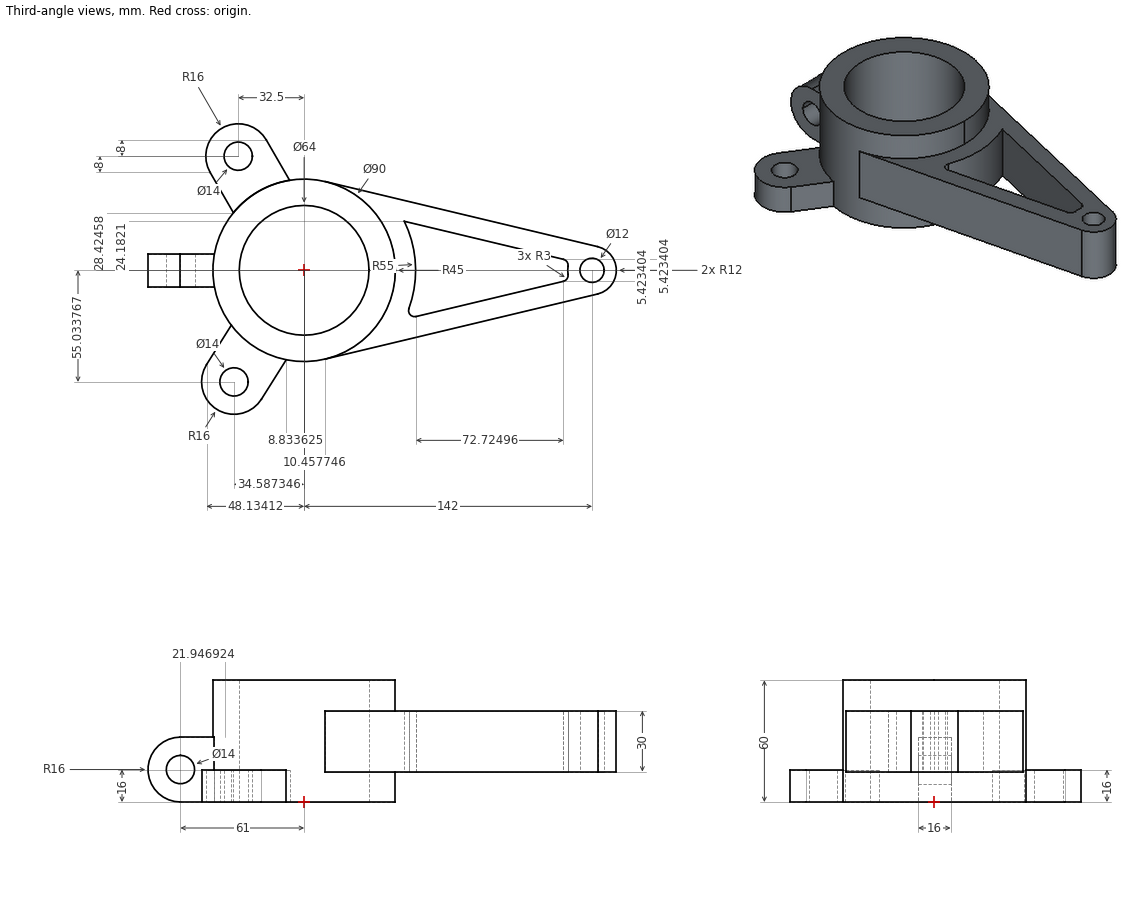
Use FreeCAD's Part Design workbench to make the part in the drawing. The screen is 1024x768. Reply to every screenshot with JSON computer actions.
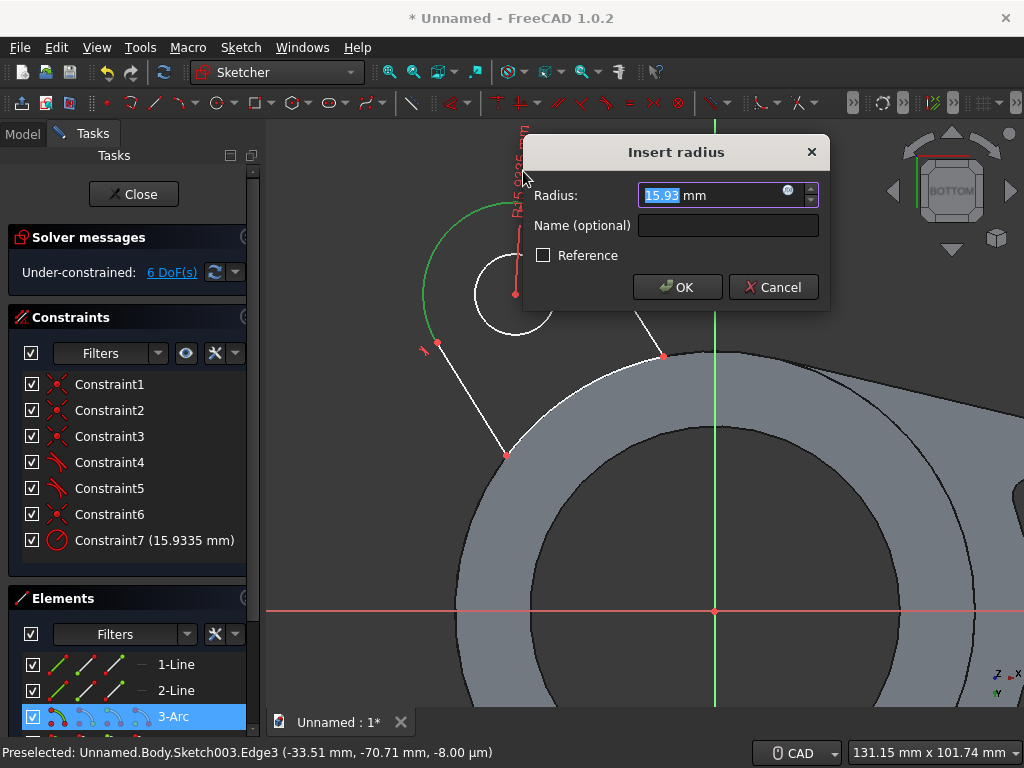
{"action": "type", "text": "16"}
{"action": "key", "text": "Return"}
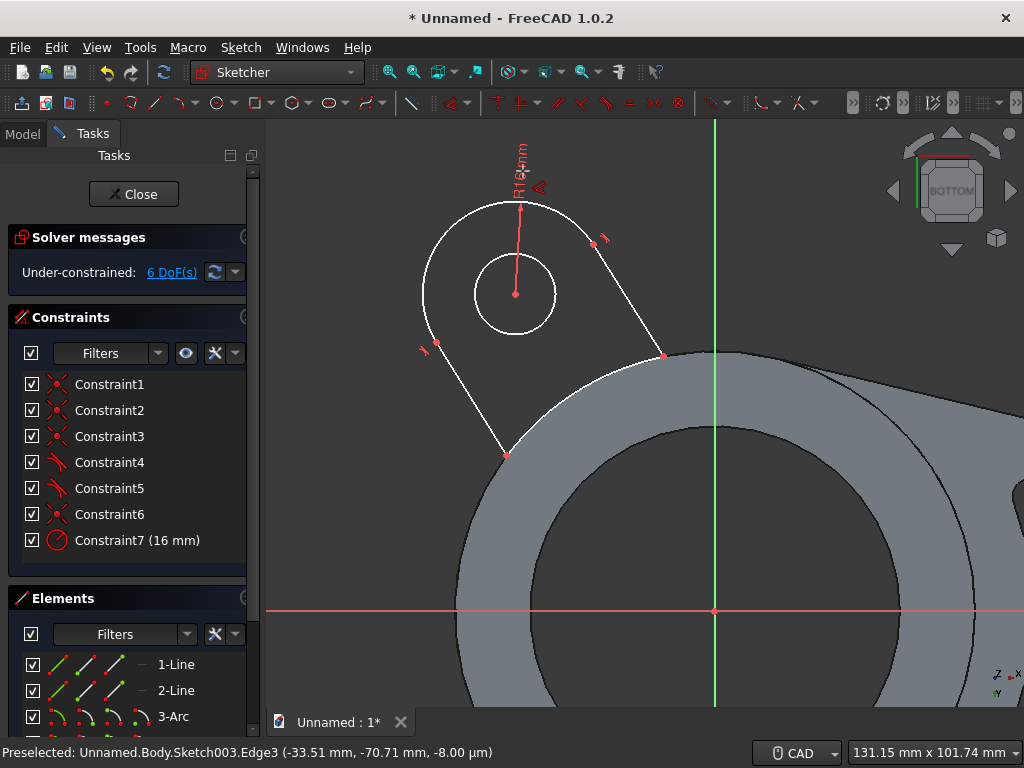
{"action": "left_click", "coordinate": [610, 374]}
{"action": "left_click", "coordinate": [597, 345]}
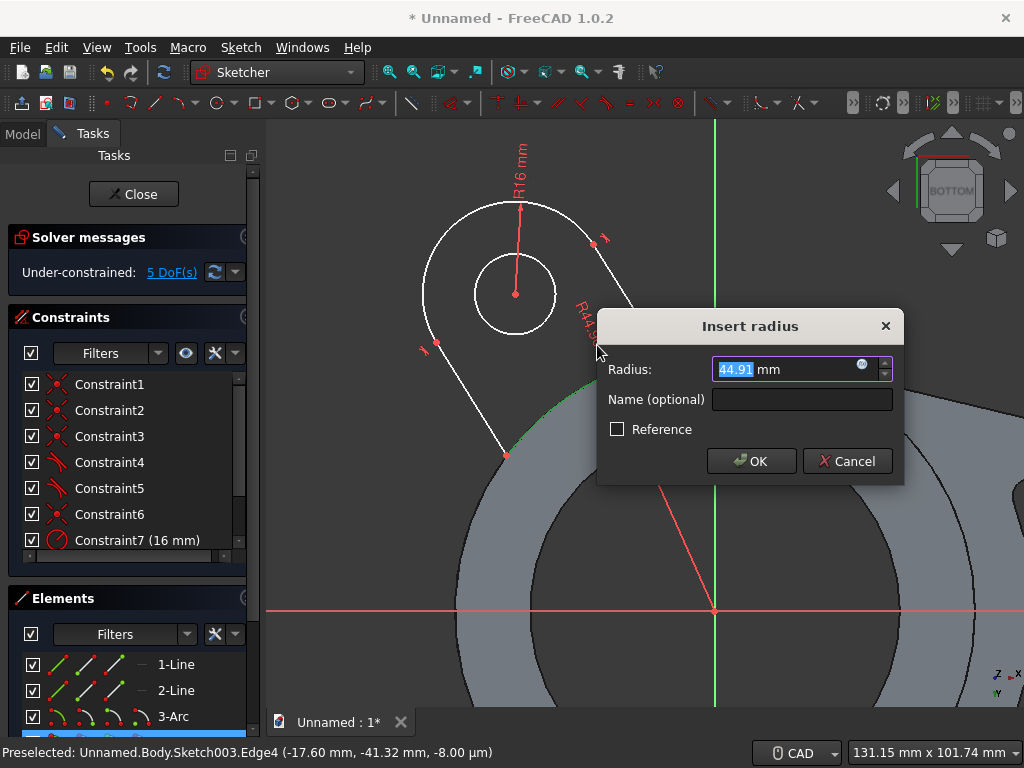
{"action": "type", "text": "45"}
{"action": "key", "text": "Return"}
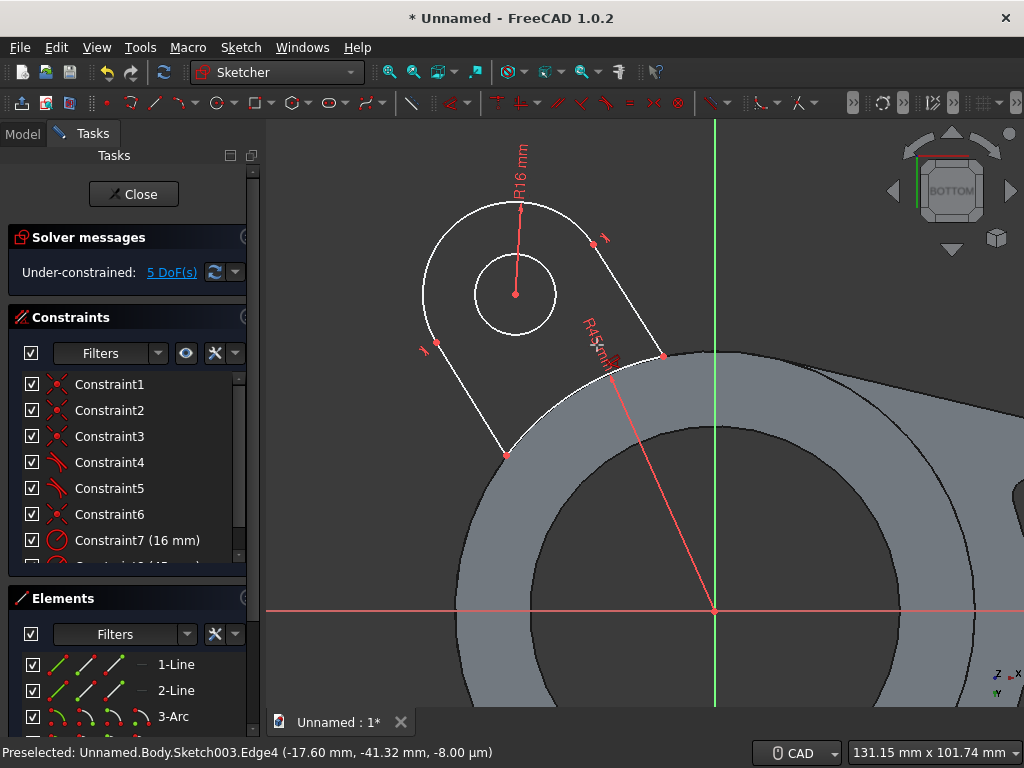
{"action": "left_click", "coordinate": [544, 266]}
{"action": "left_click", "coordinate": [567, 243]}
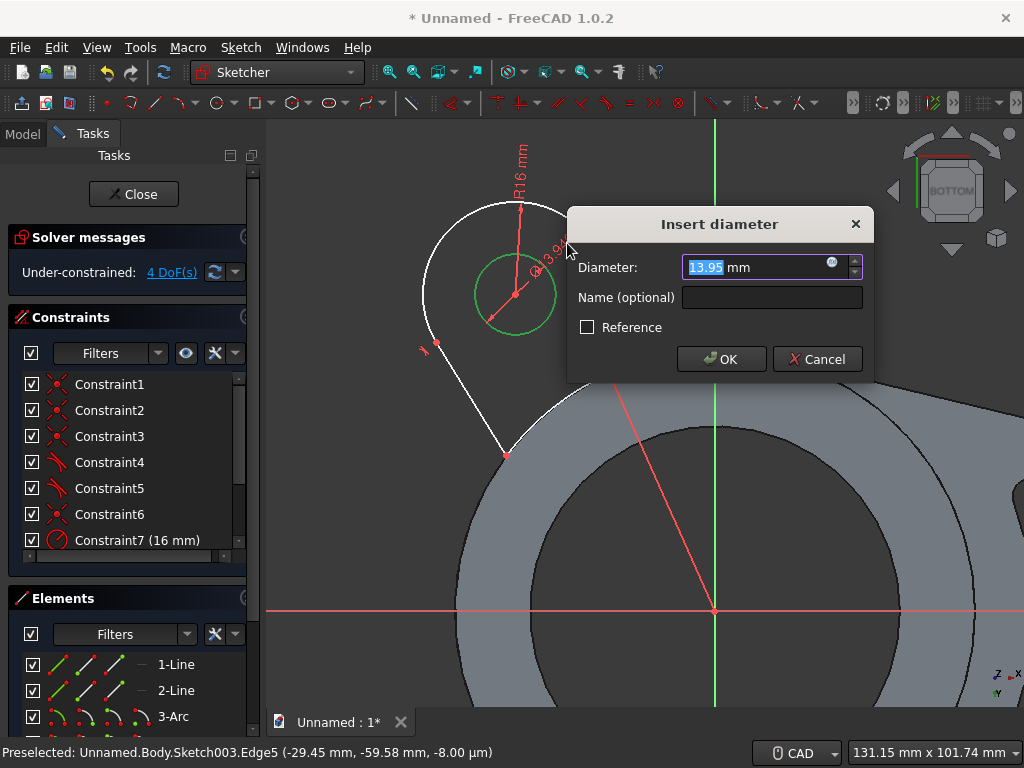
{"action": "type", "text": "14"}
{"action": "key", "text": "Return"}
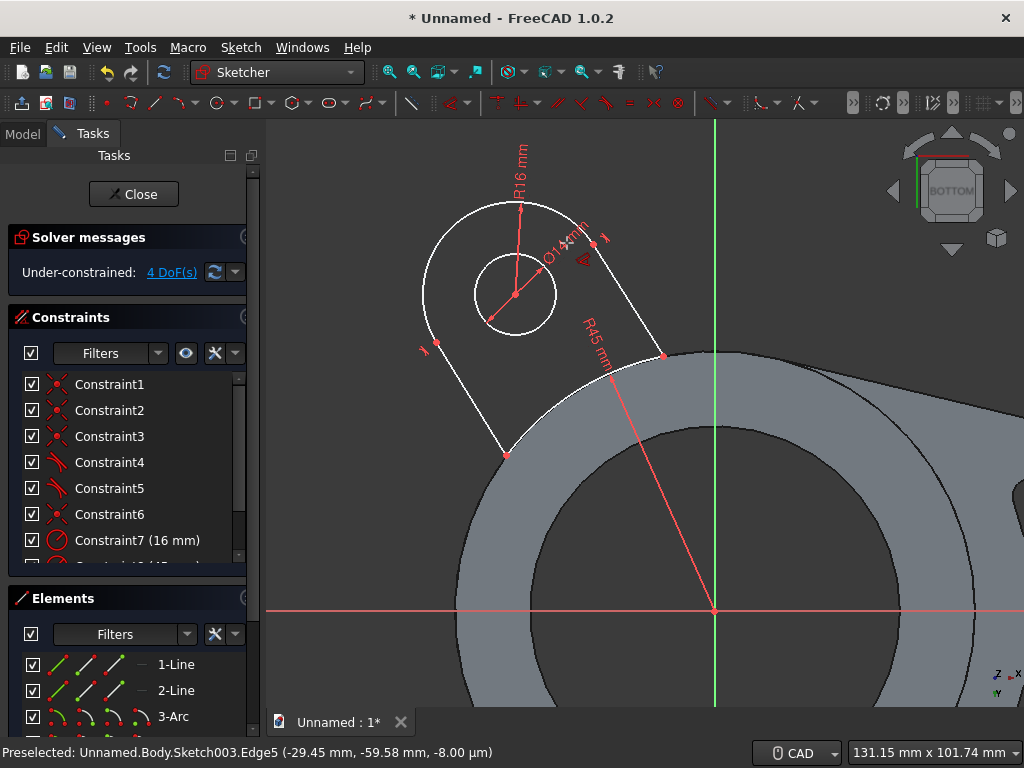
{"action": "left_click", "coordinate": [437, 343]}
{"action": "left_click", "coordinate": [576, 645]}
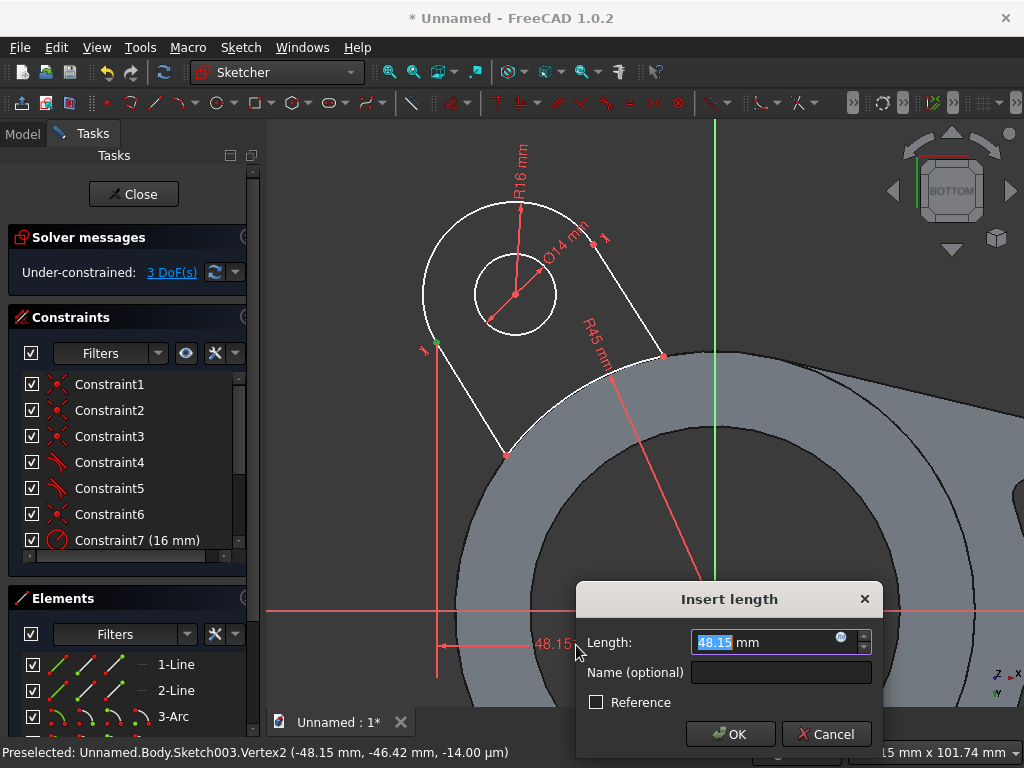
{"action": "type", "text": "48.13412"}
{"action": "key", "text": "Return"}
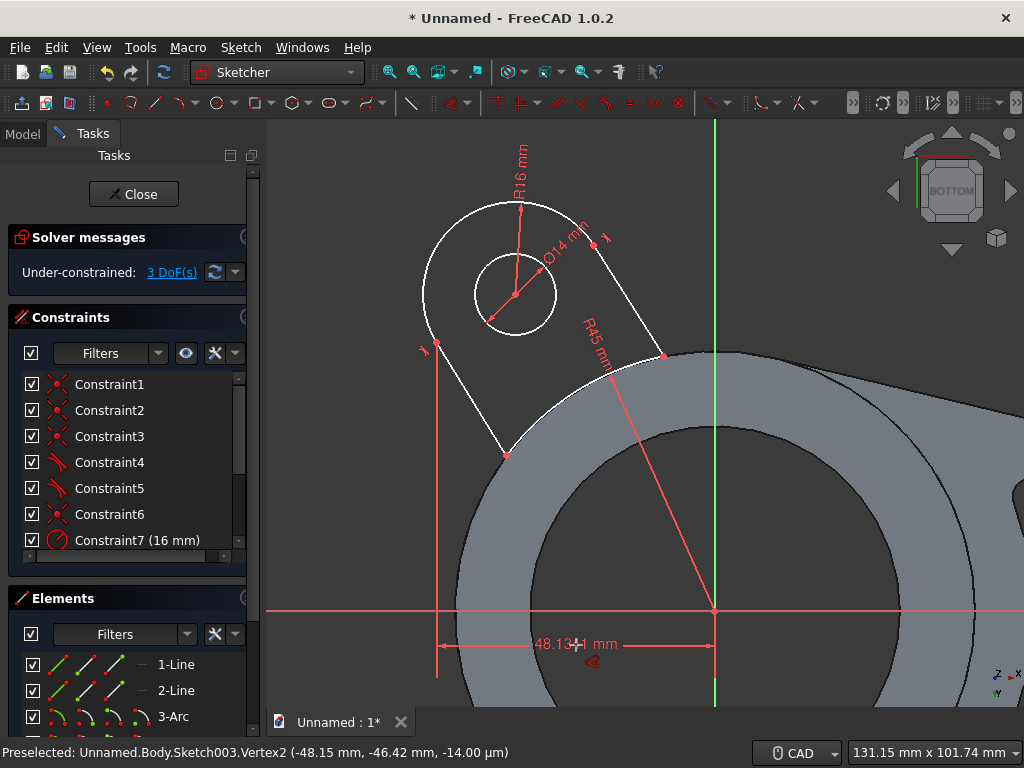
{"action": "left_click", "coordinate": [664, 356]}
{"action": "left_click", "coordinate": [689, 645]}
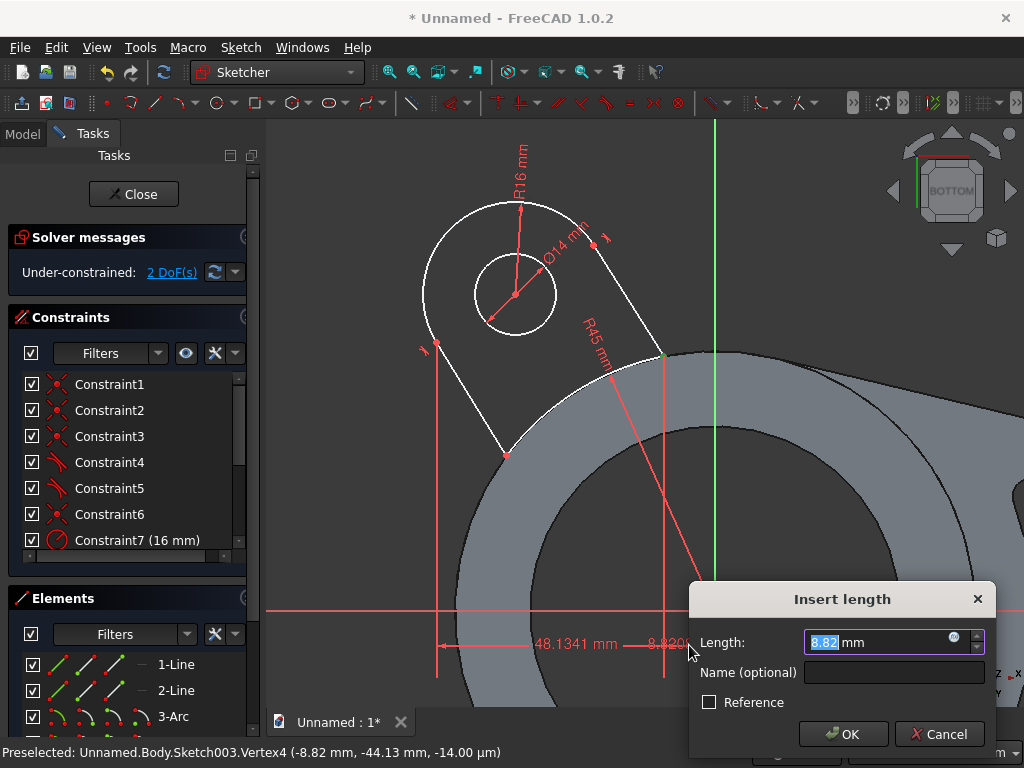
{"action": "type", "text": "8.833625"}
{"action": "key", "text": "Return"}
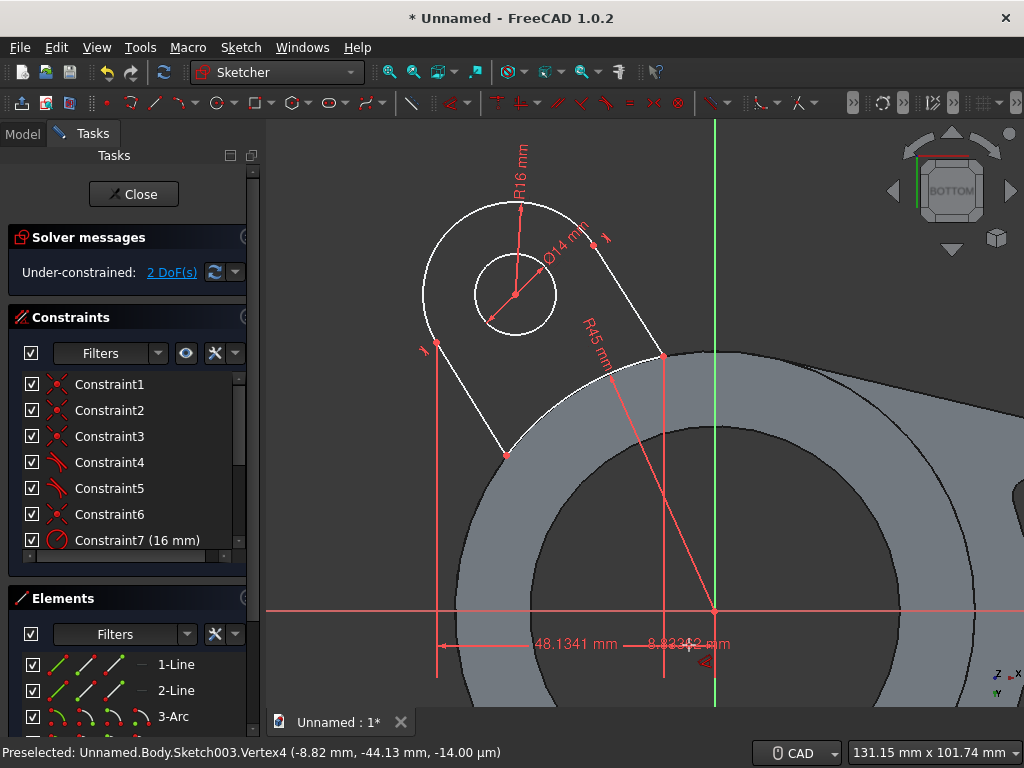
{"action": "left_click", "coordinate": [516, 295]}
{"action": "left_click", "coordinate": [661, 261]}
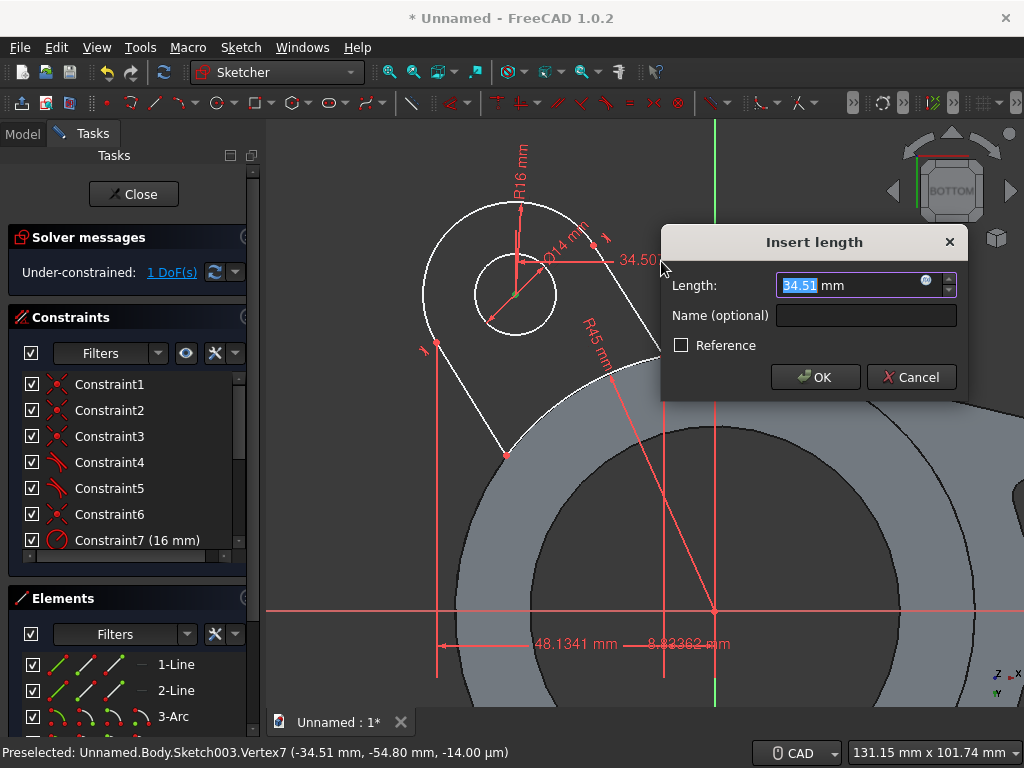
{"action": "type", "text": "34.587346"}
{"action": "key", "text": "Return"}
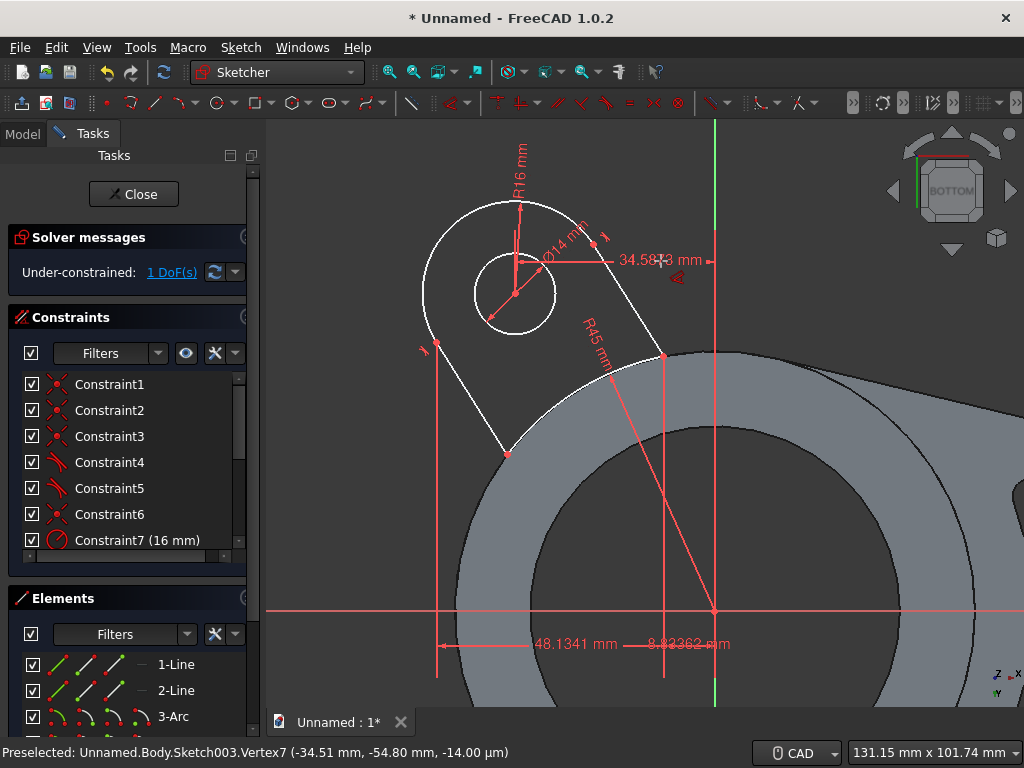
{"action": "left_click", "coordinate": [515, 294]}
{"action": "left_click", "coordinate": [749, 453]}